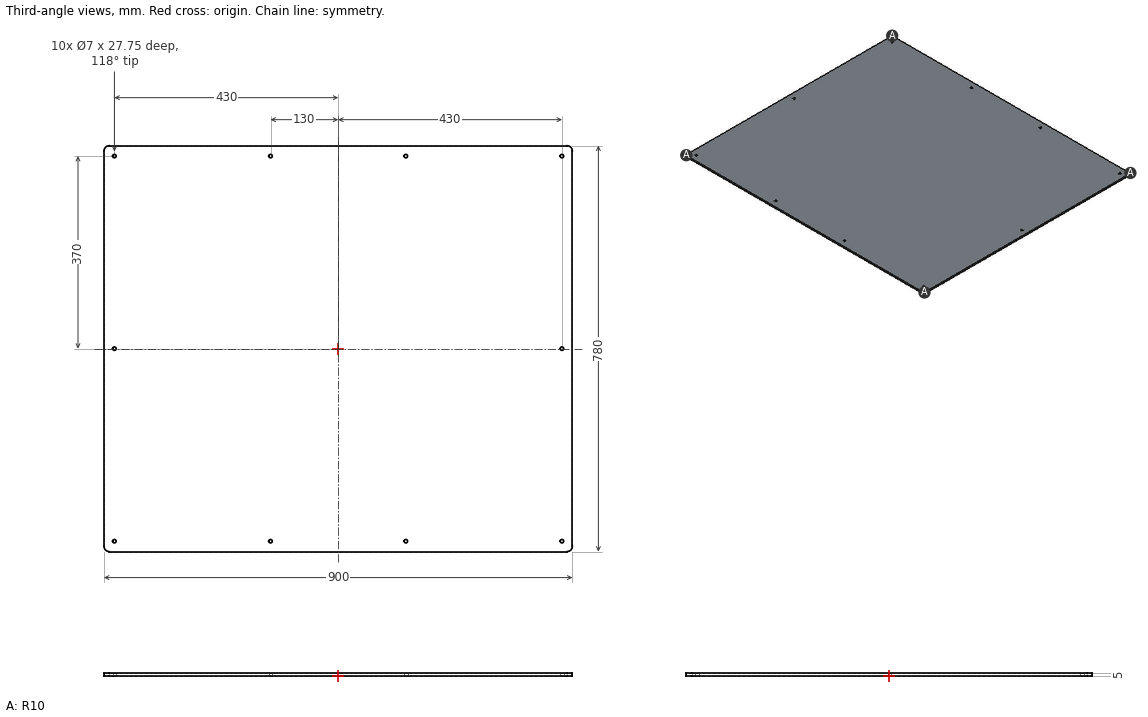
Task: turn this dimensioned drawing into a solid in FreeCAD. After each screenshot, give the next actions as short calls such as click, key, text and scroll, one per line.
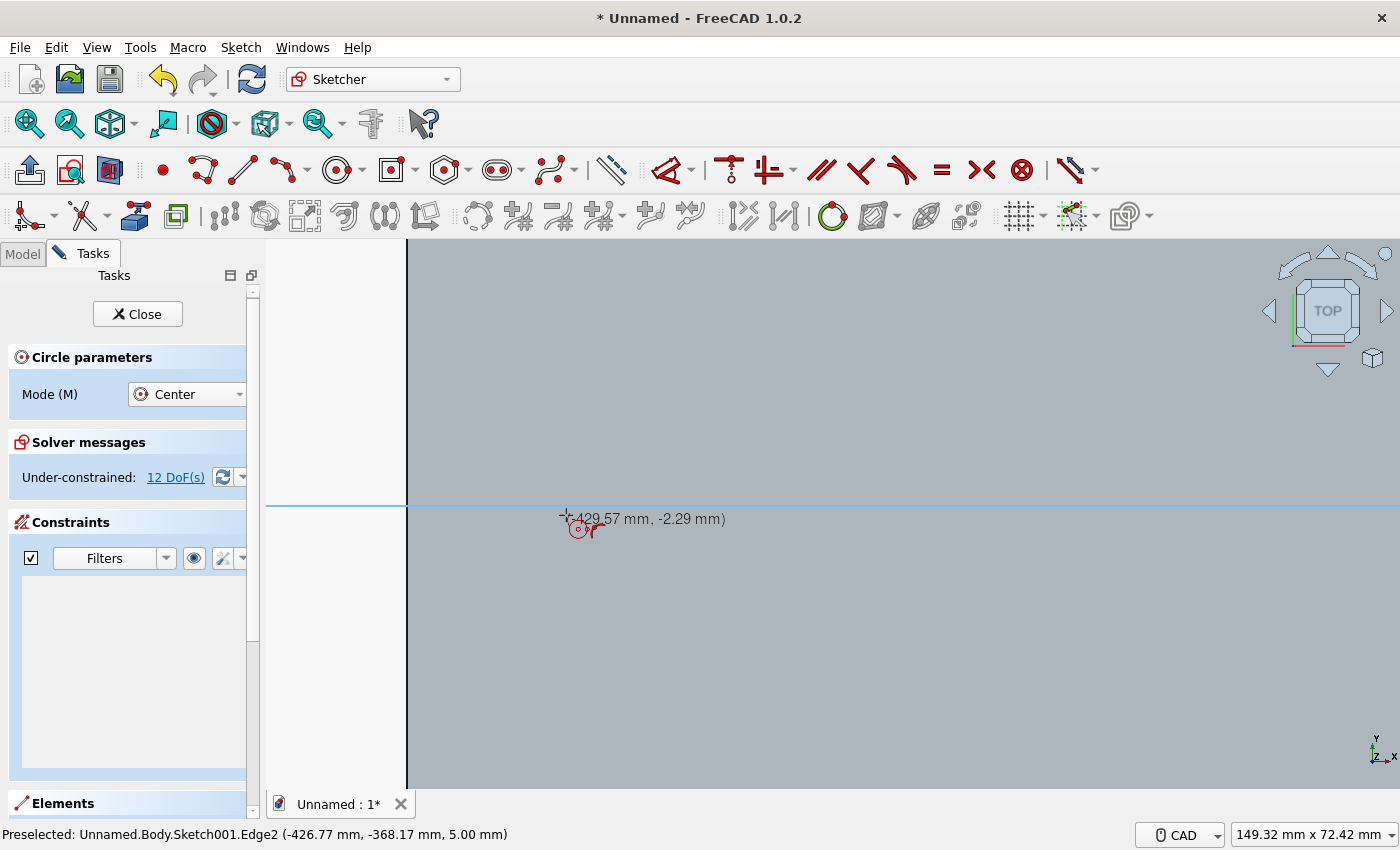
scroll(566, 515, down, 14)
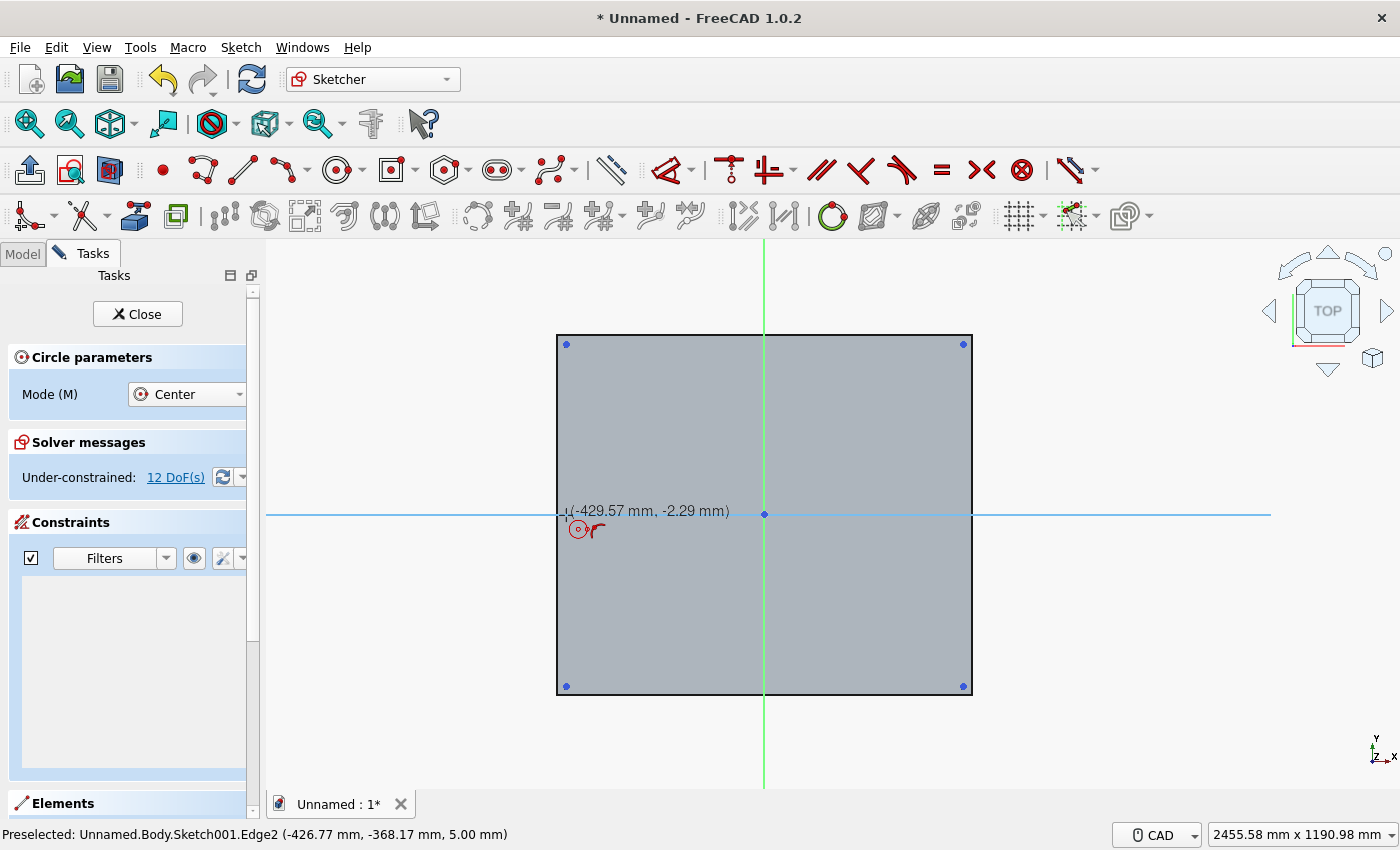
click(566, 515)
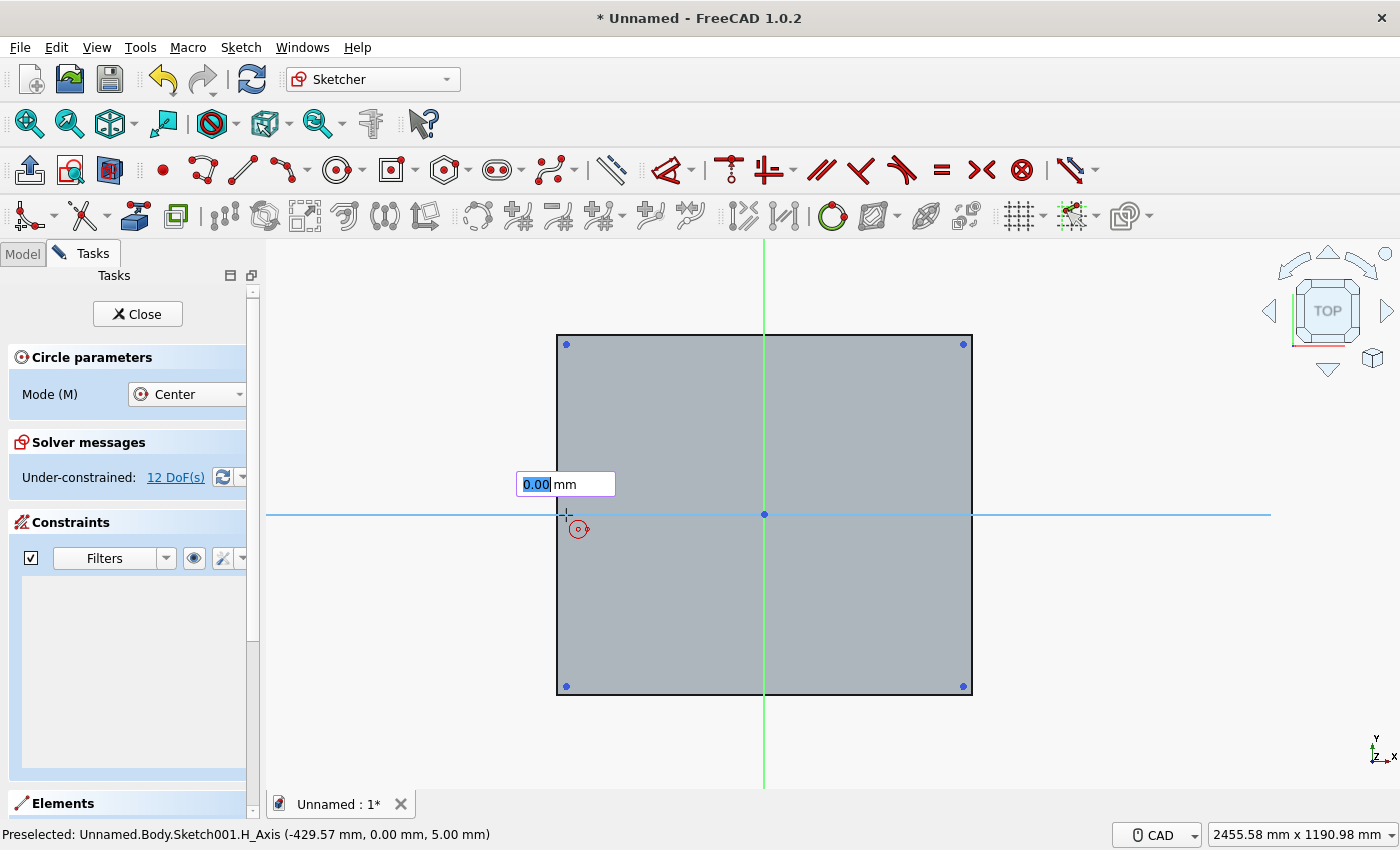
scroll(566, 513, up, 12)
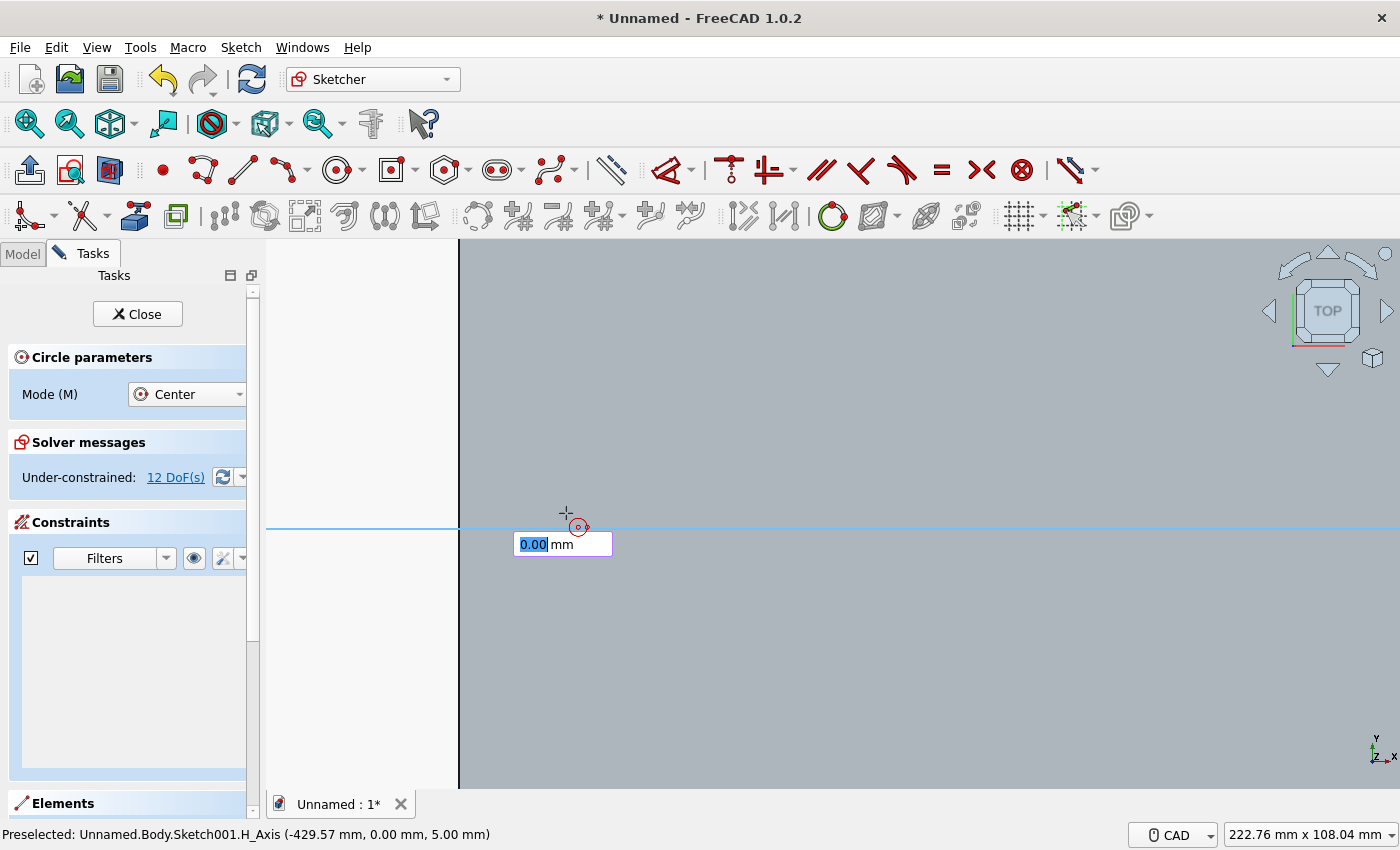
click(567, 513)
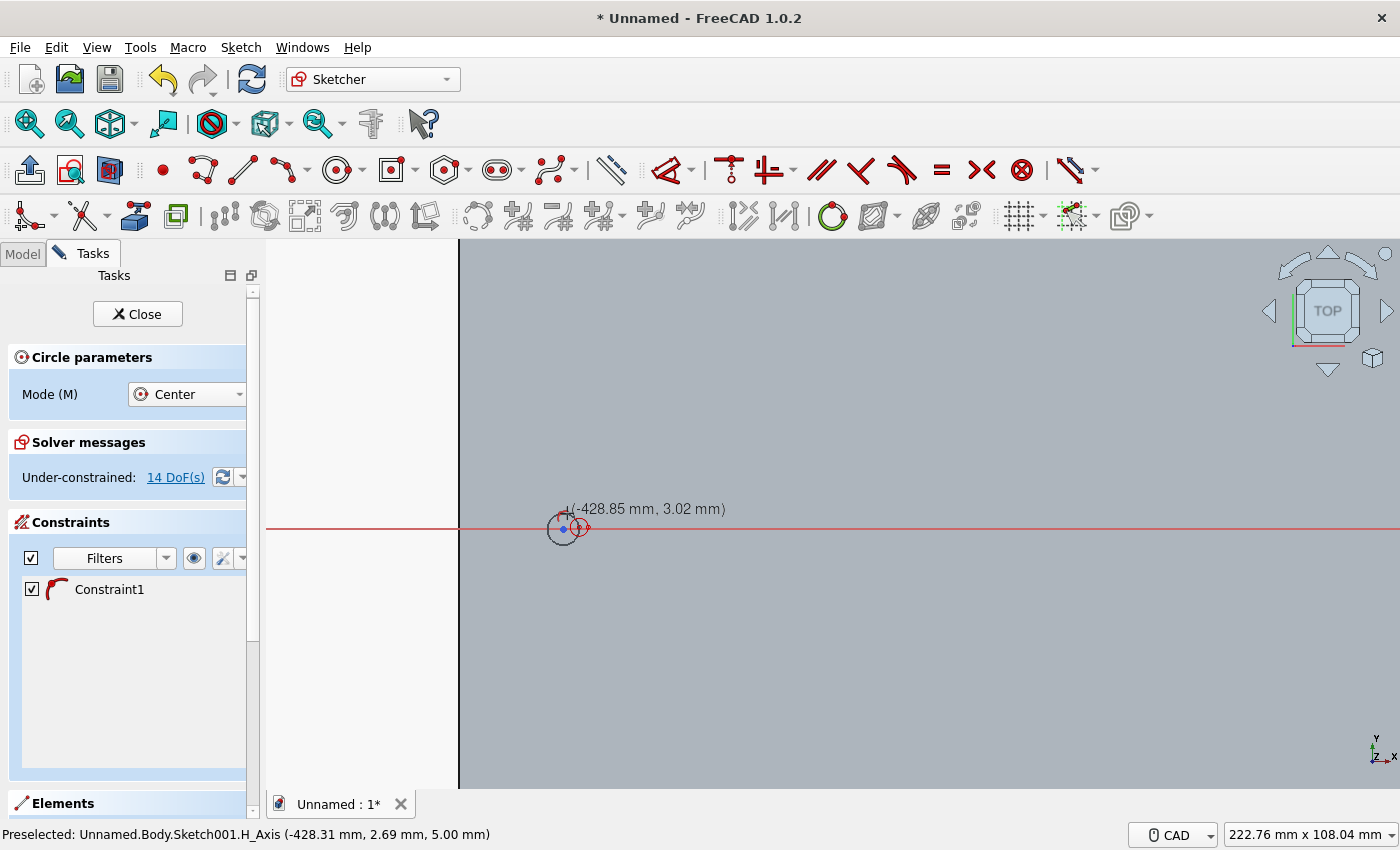
scroll(566, 512, down, 12)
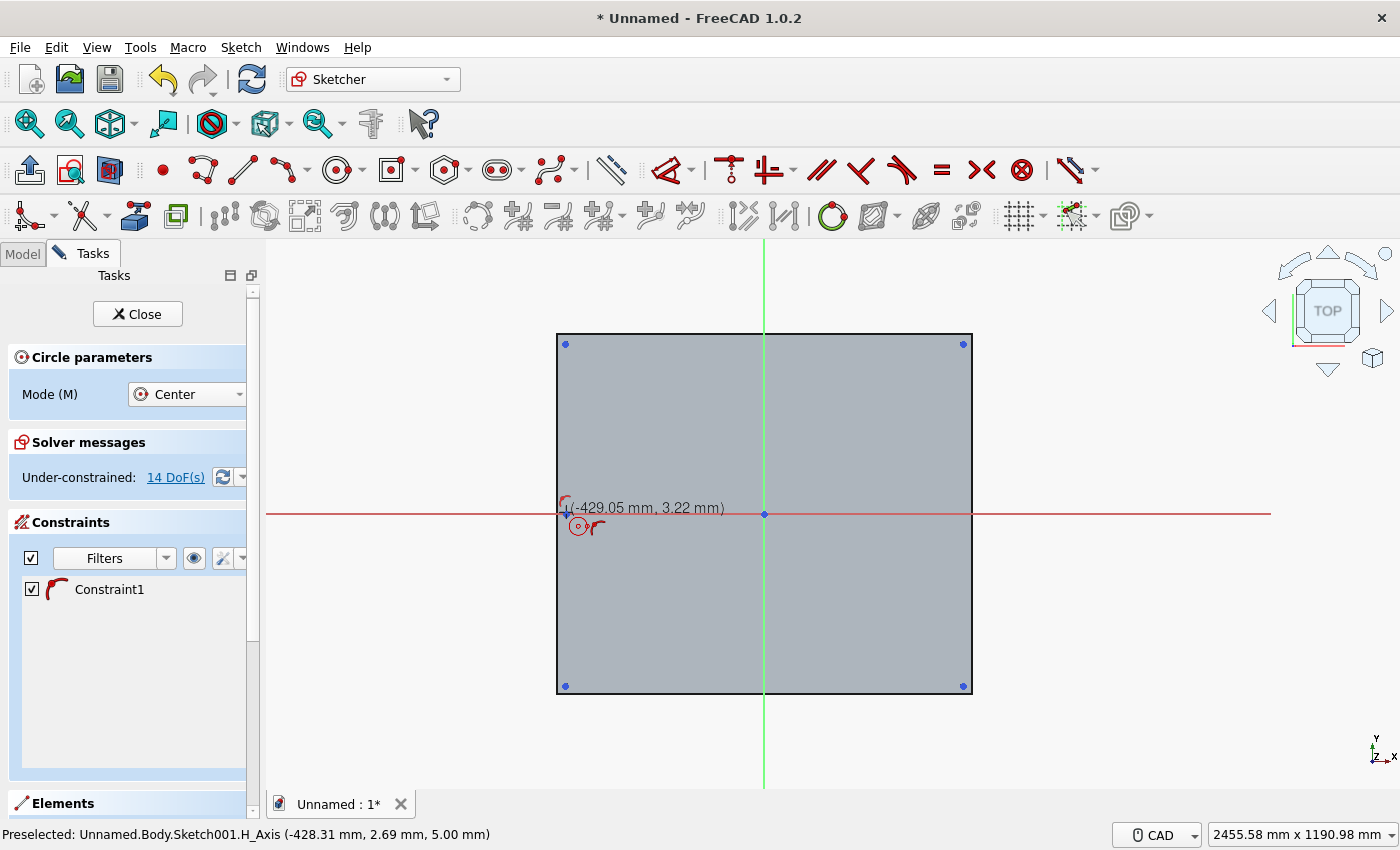
scroll(963, 514, up, 14)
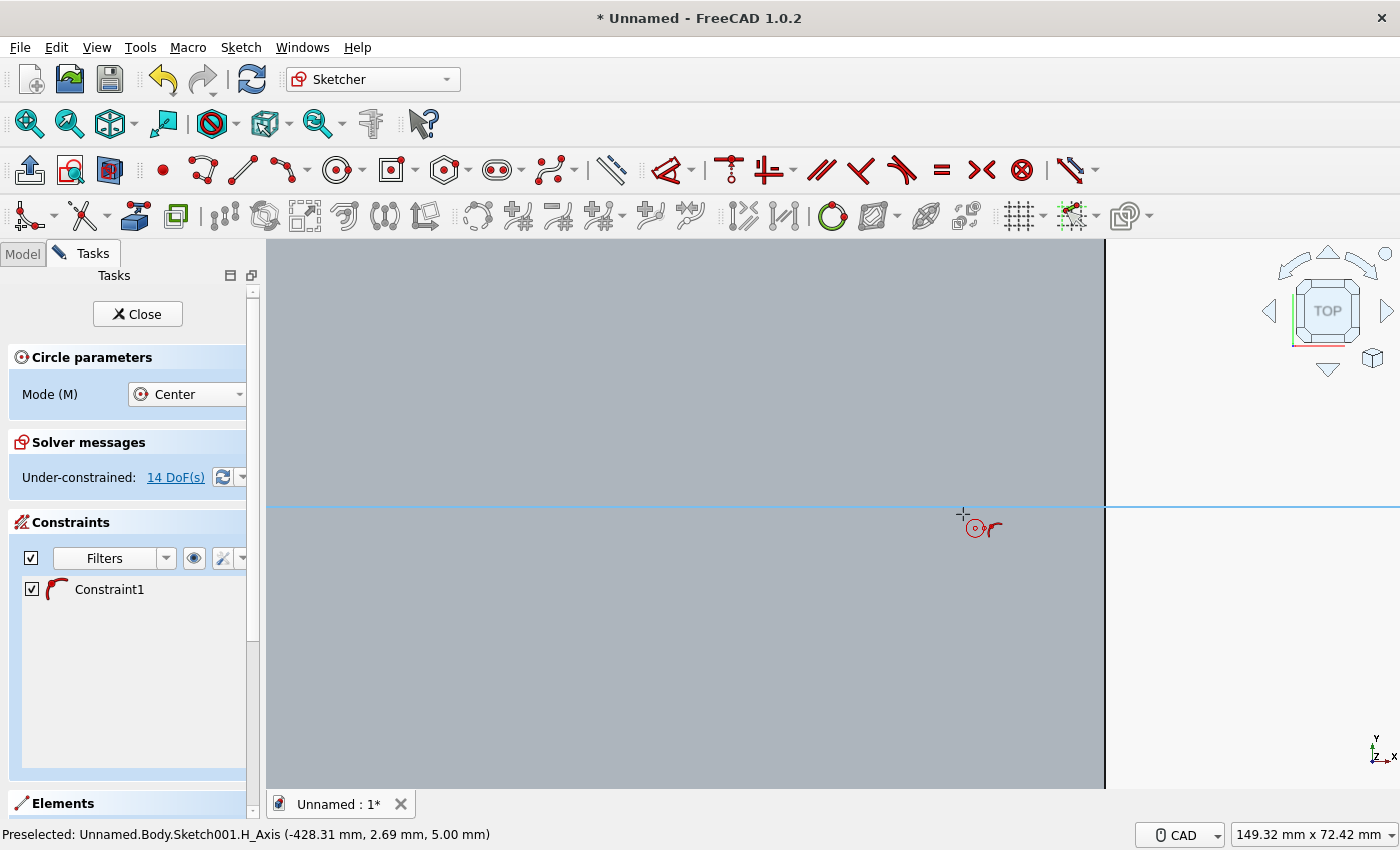
scroll(964, 514, down, 14)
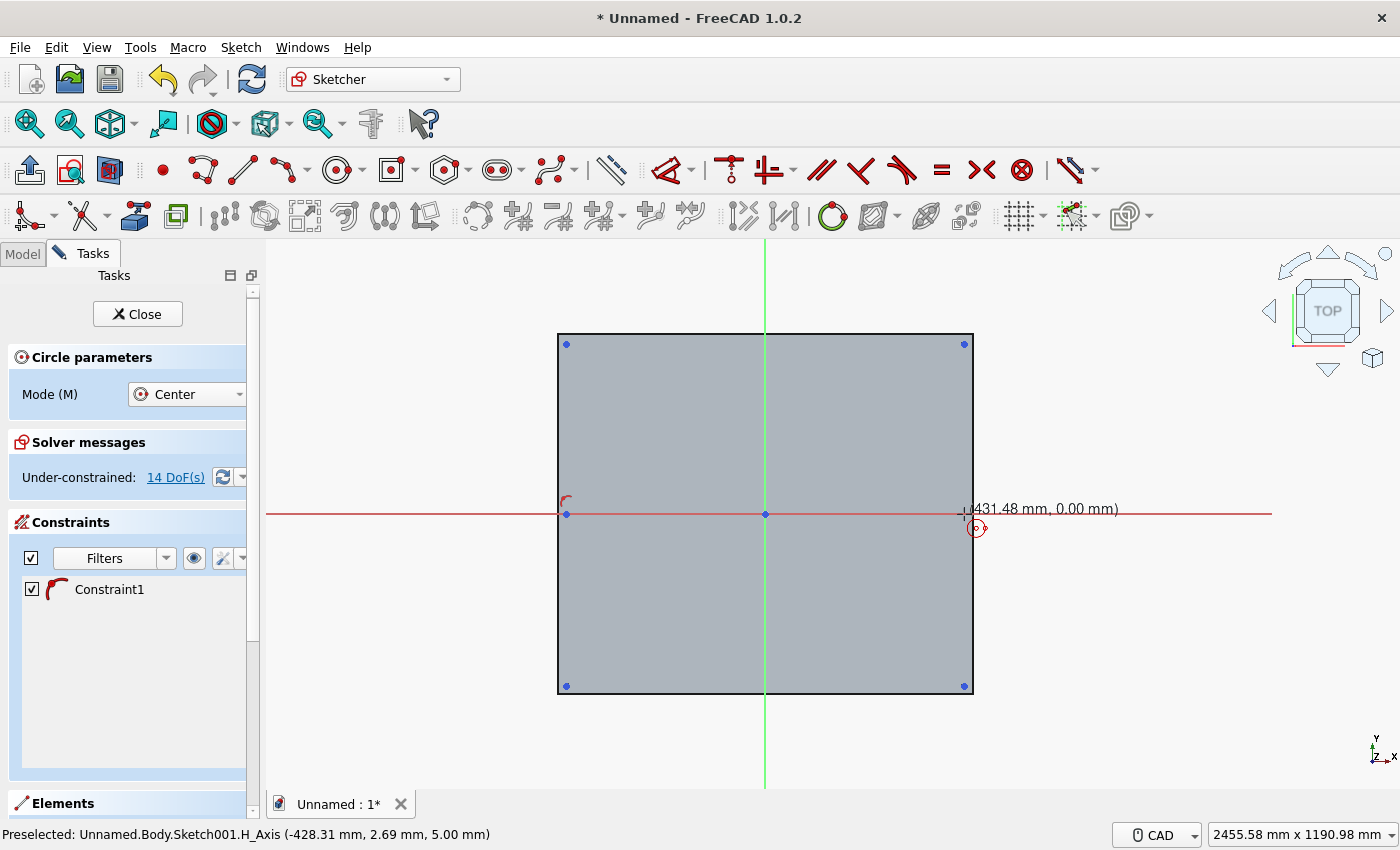
click(964, 514)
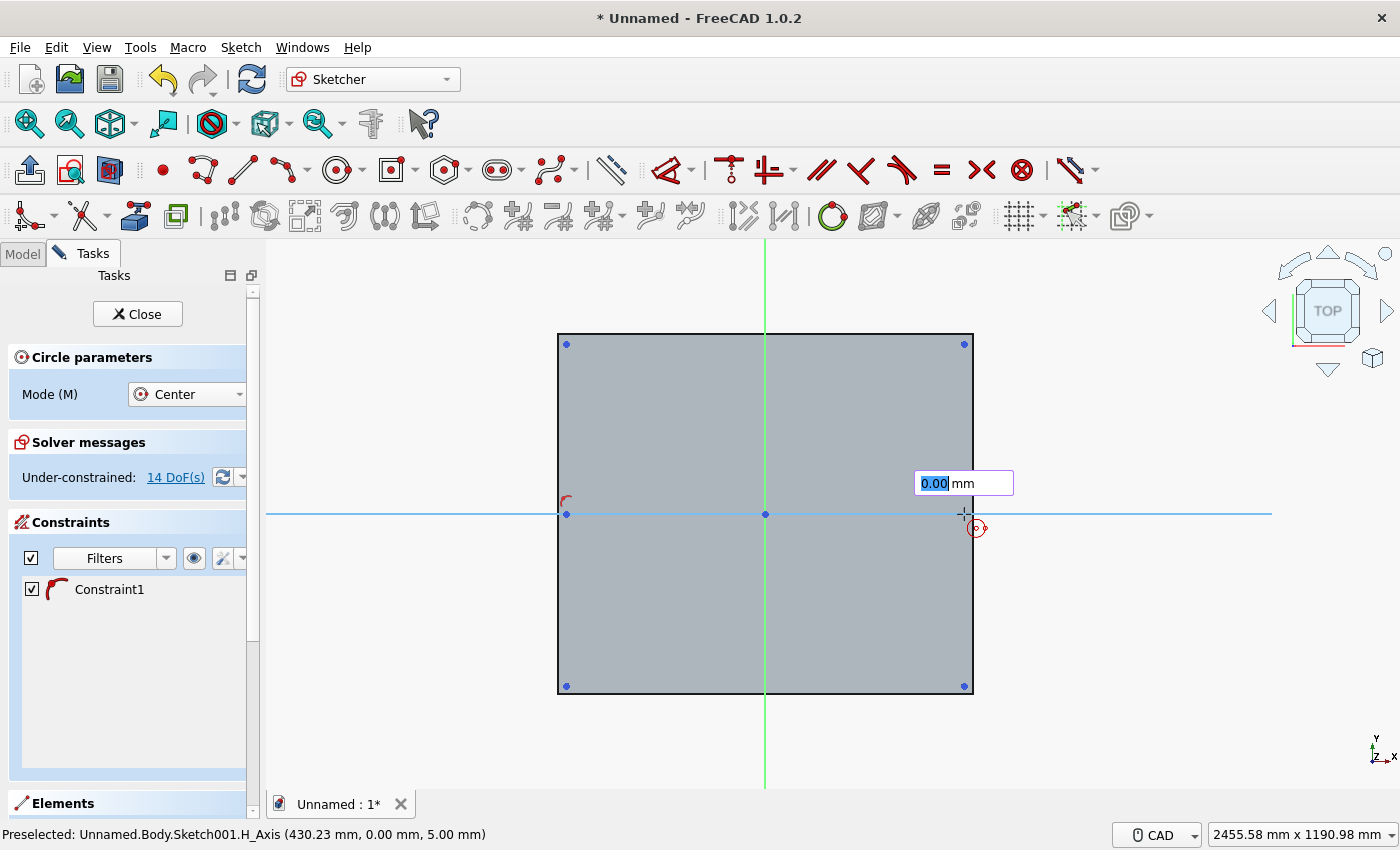
scroll(964, 513, up, 12)